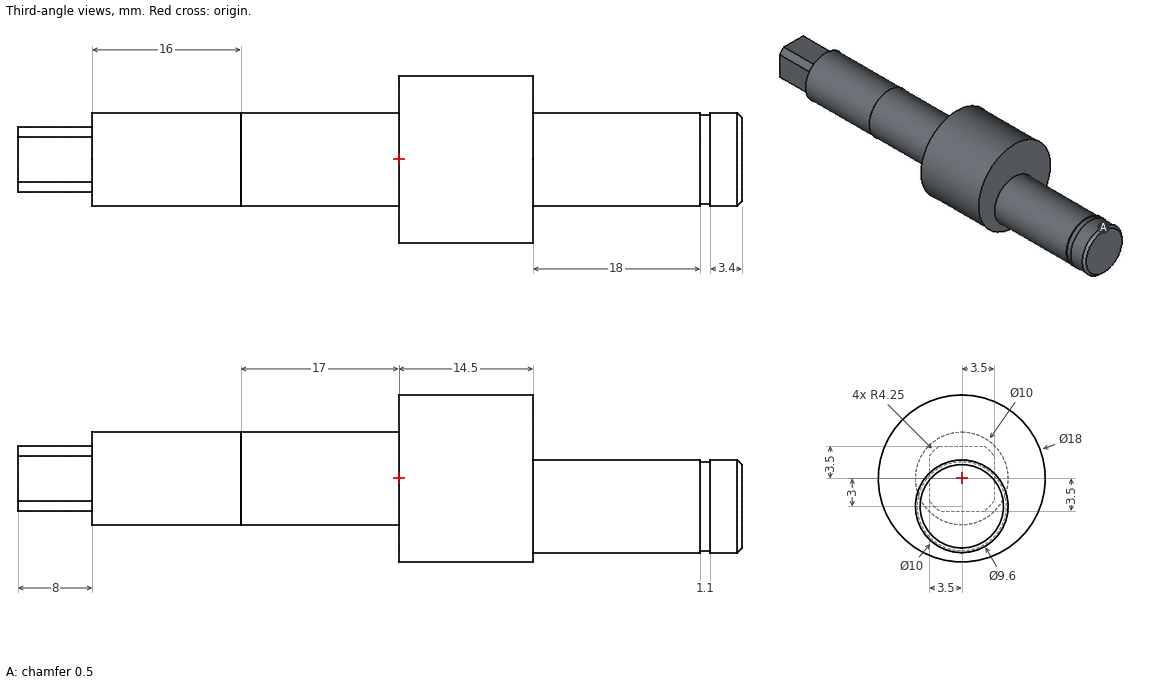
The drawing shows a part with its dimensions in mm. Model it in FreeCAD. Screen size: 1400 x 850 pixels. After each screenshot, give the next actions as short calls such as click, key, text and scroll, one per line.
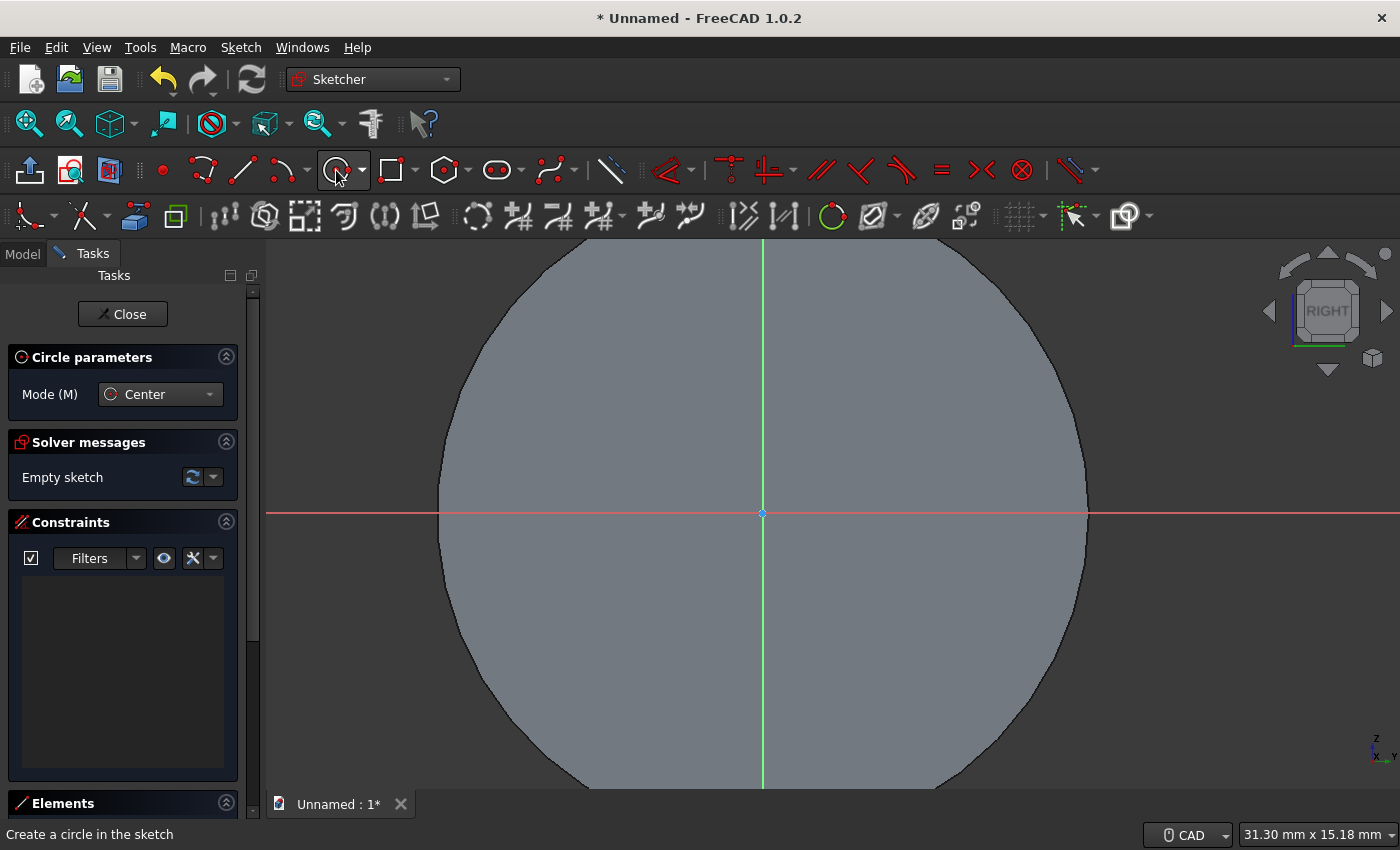
click(763, 513)
move(891, 385)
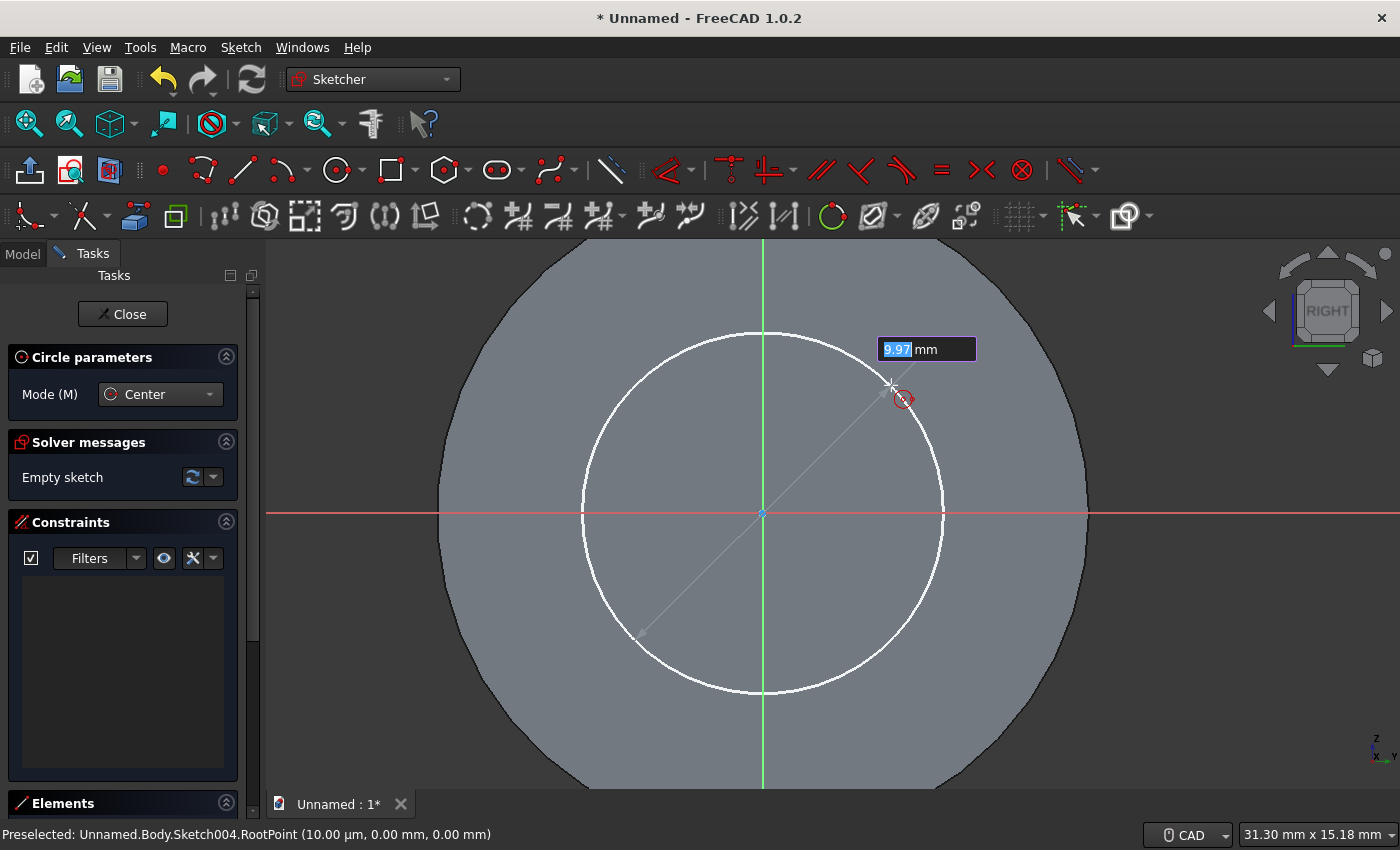
text(10)
key(Return)
key(Escape)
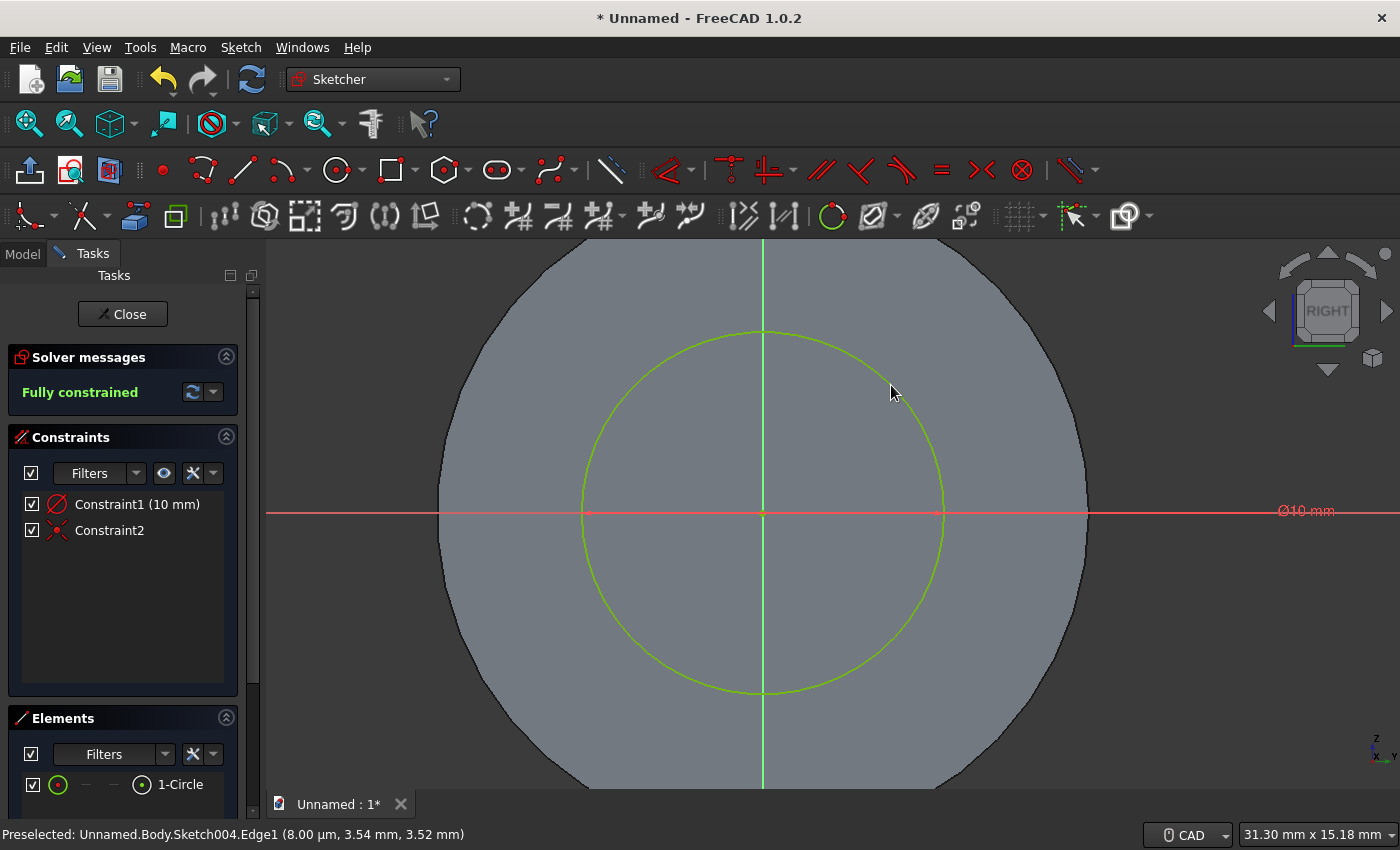
click(123, 314)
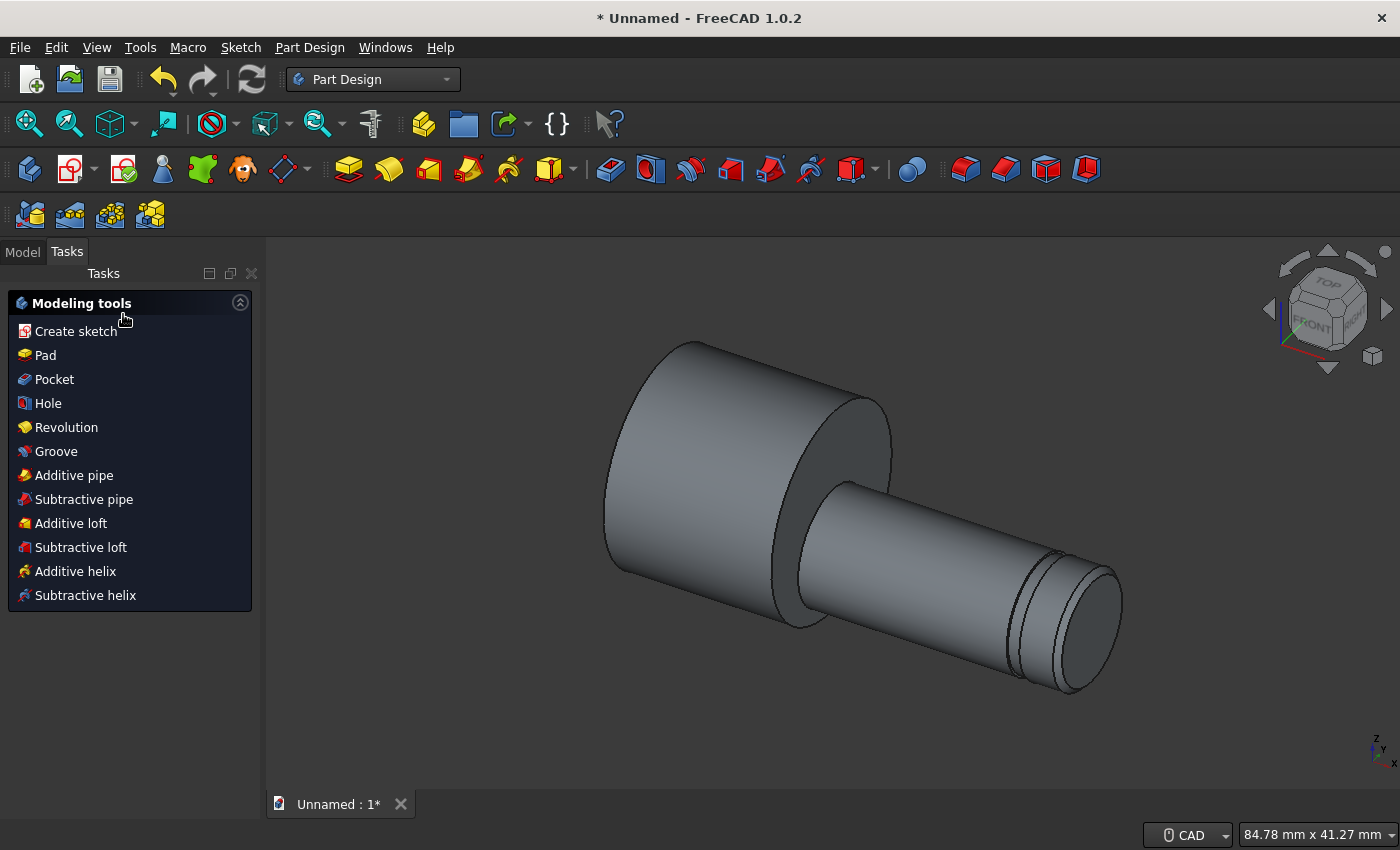
click(350, 170)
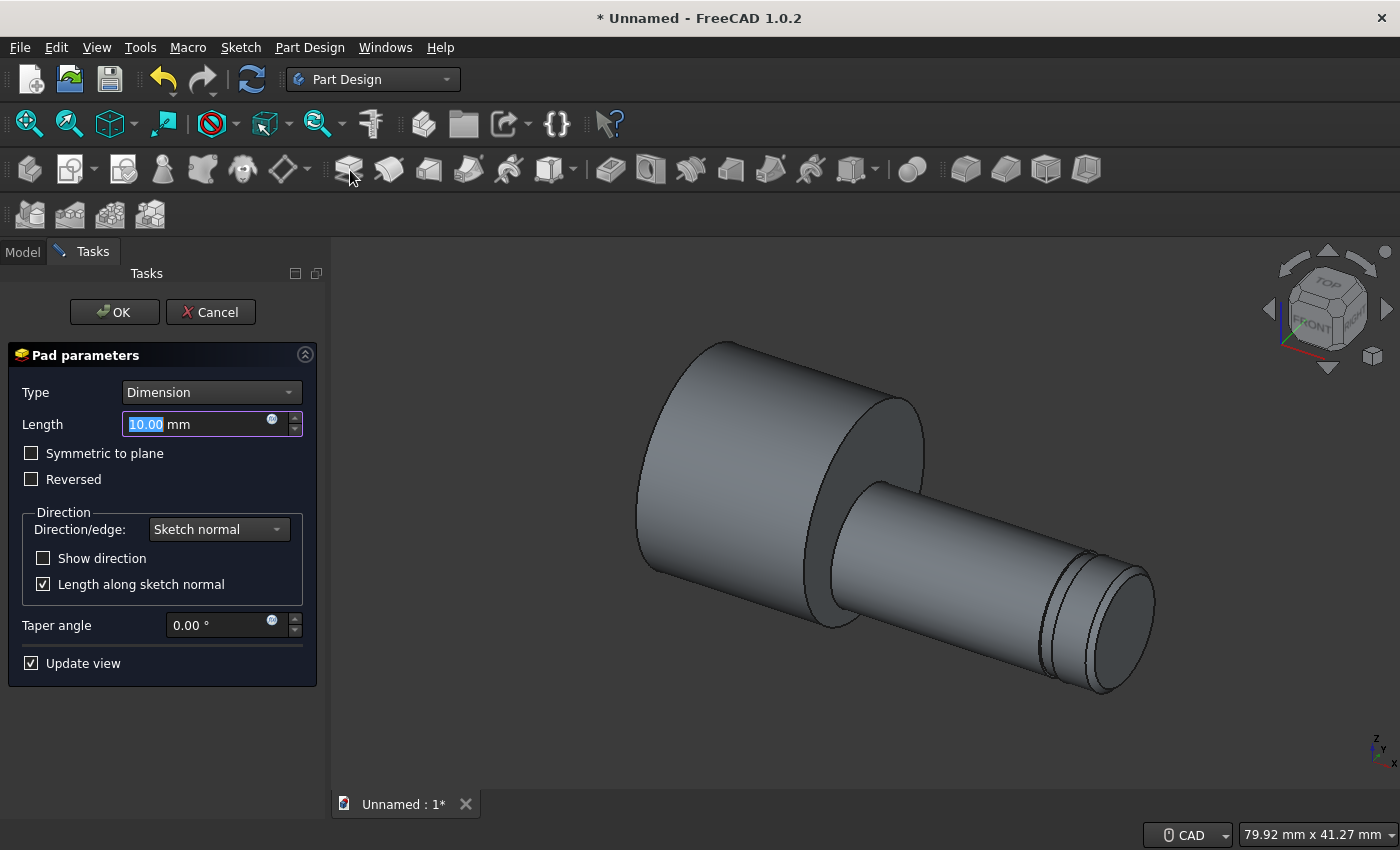
text(17)
key(Tab)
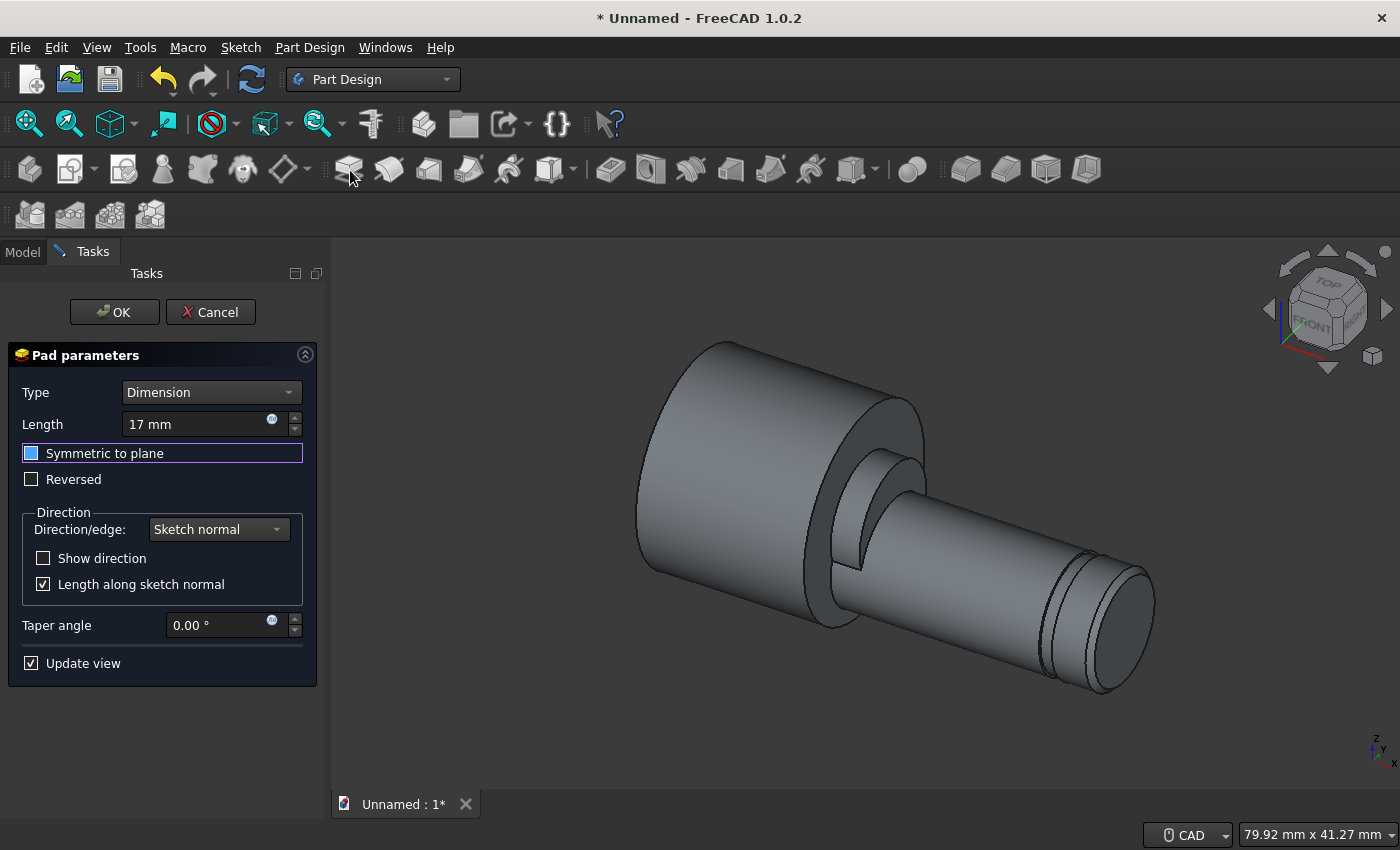
click(30, 479)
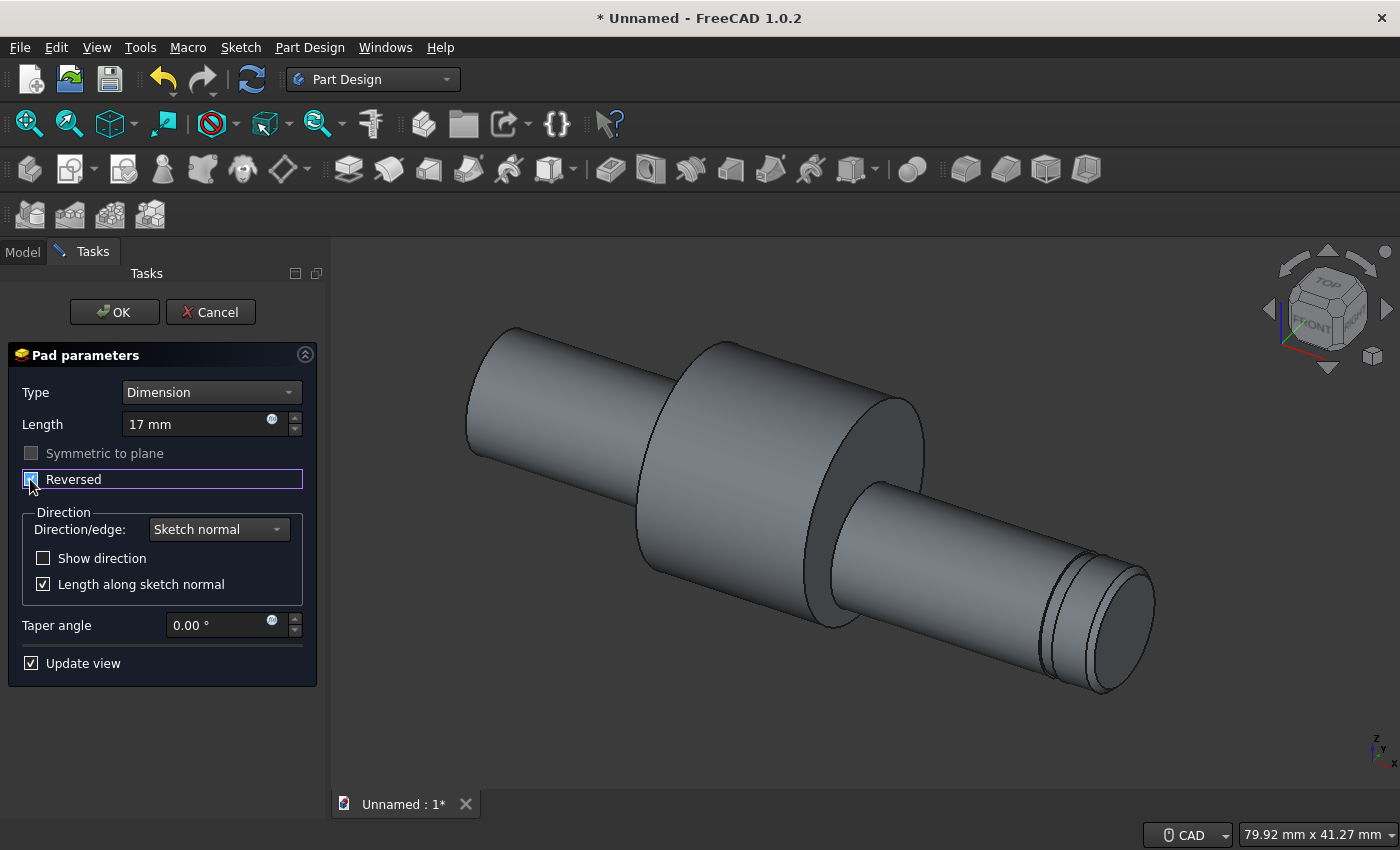
click(115, 312)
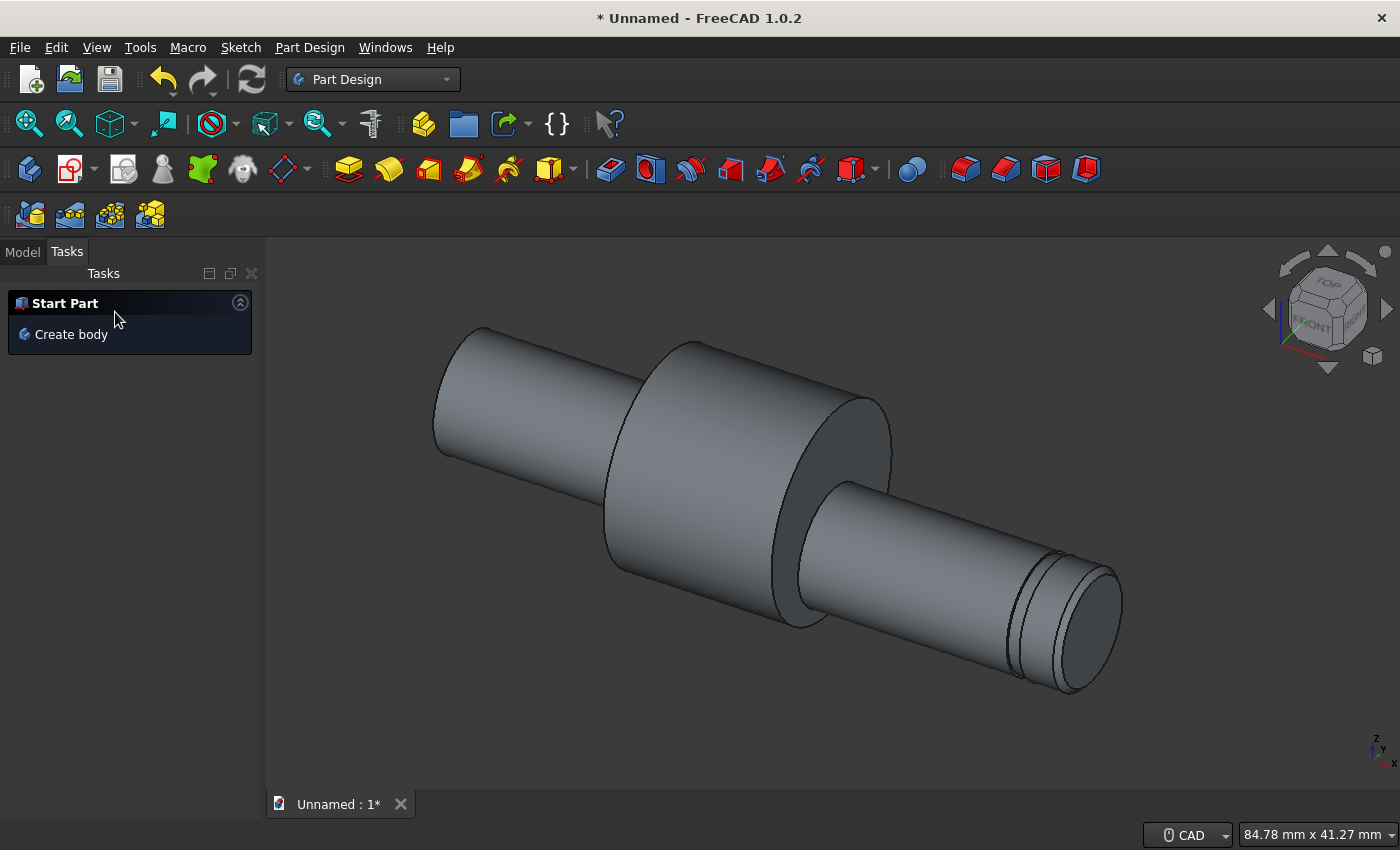
click(30, 124)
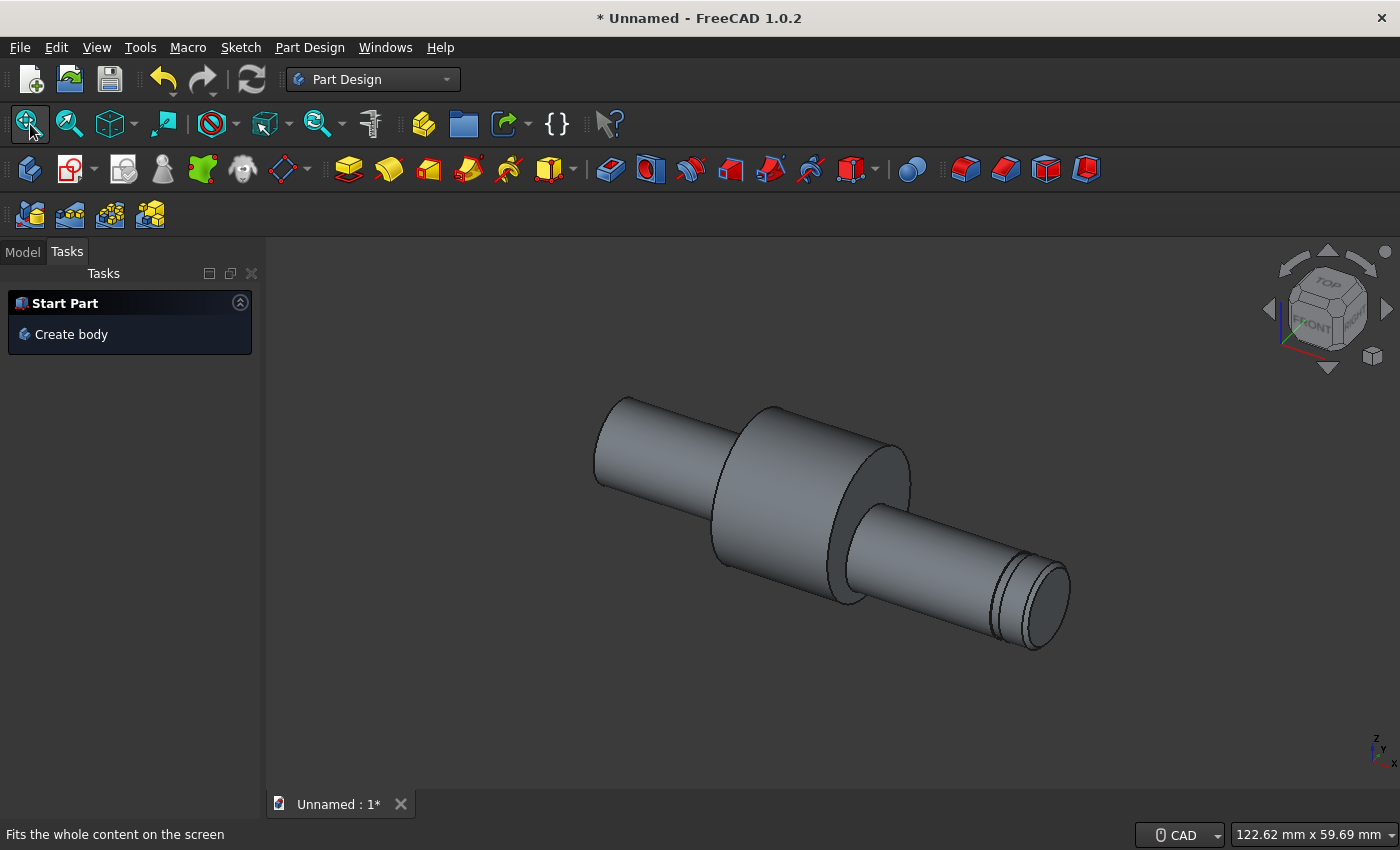
click(30, 170)